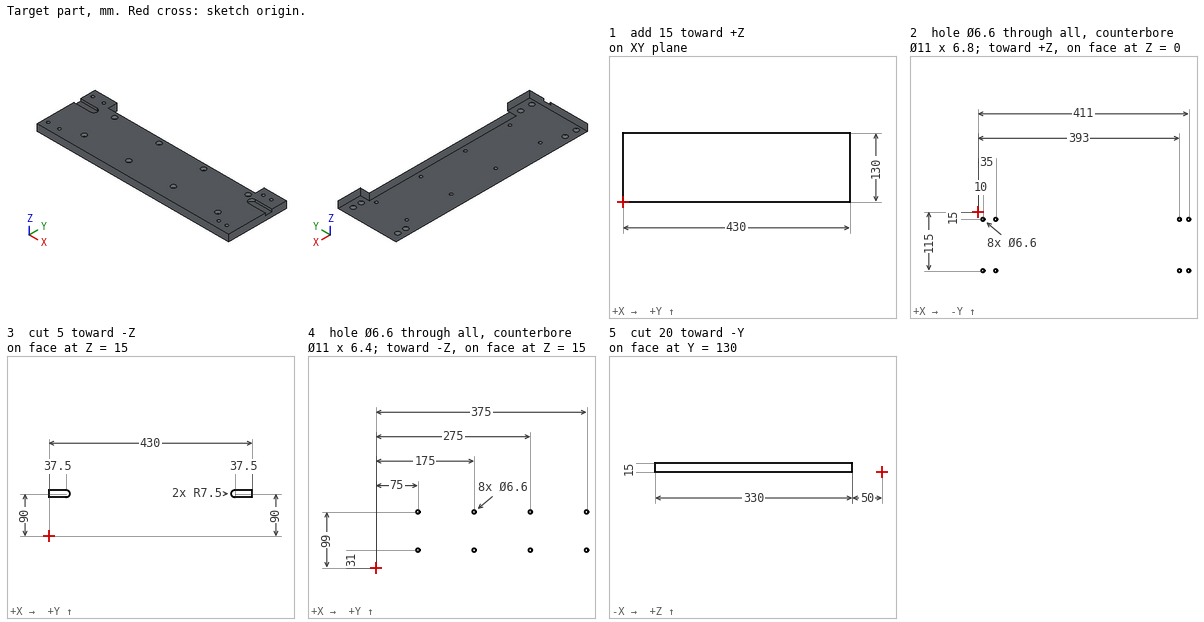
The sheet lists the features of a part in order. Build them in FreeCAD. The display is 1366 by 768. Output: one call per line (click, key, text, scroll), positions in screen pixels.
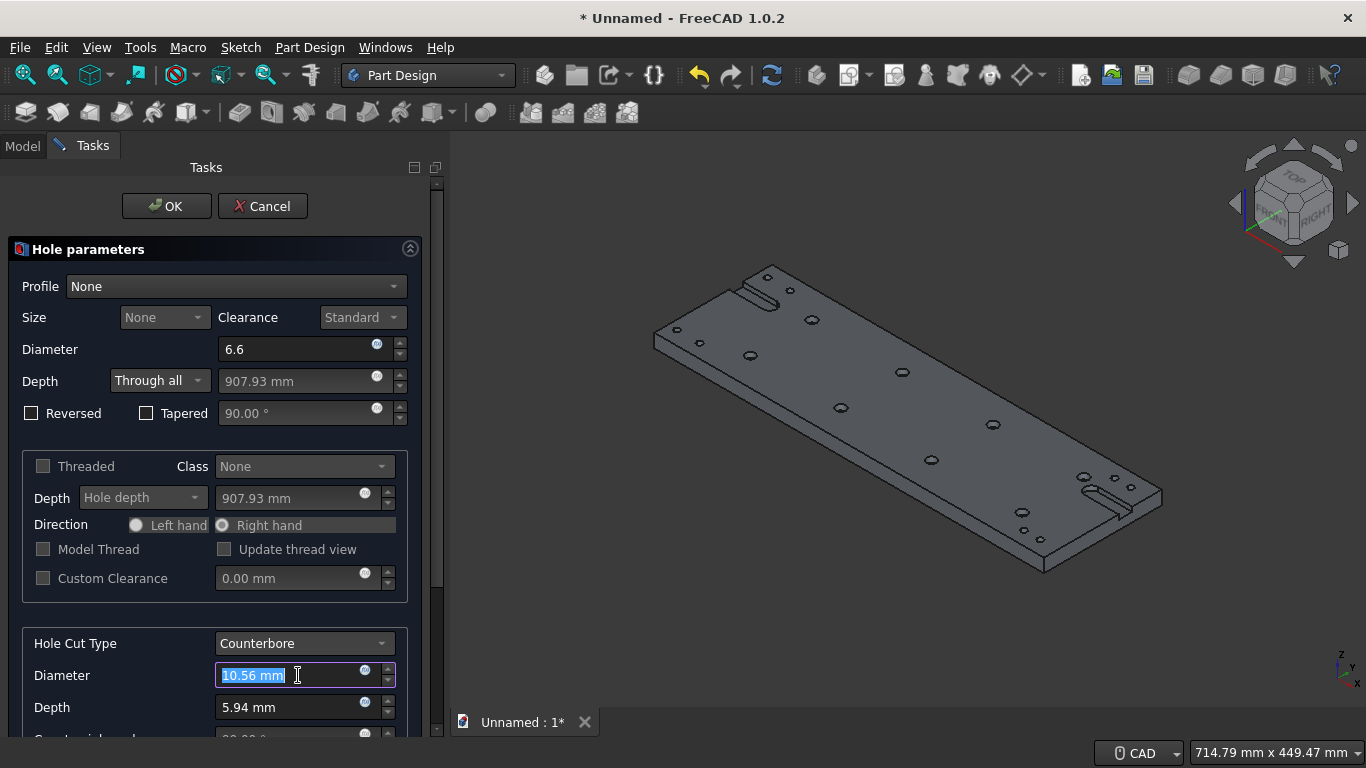
text(11)
key(Tab)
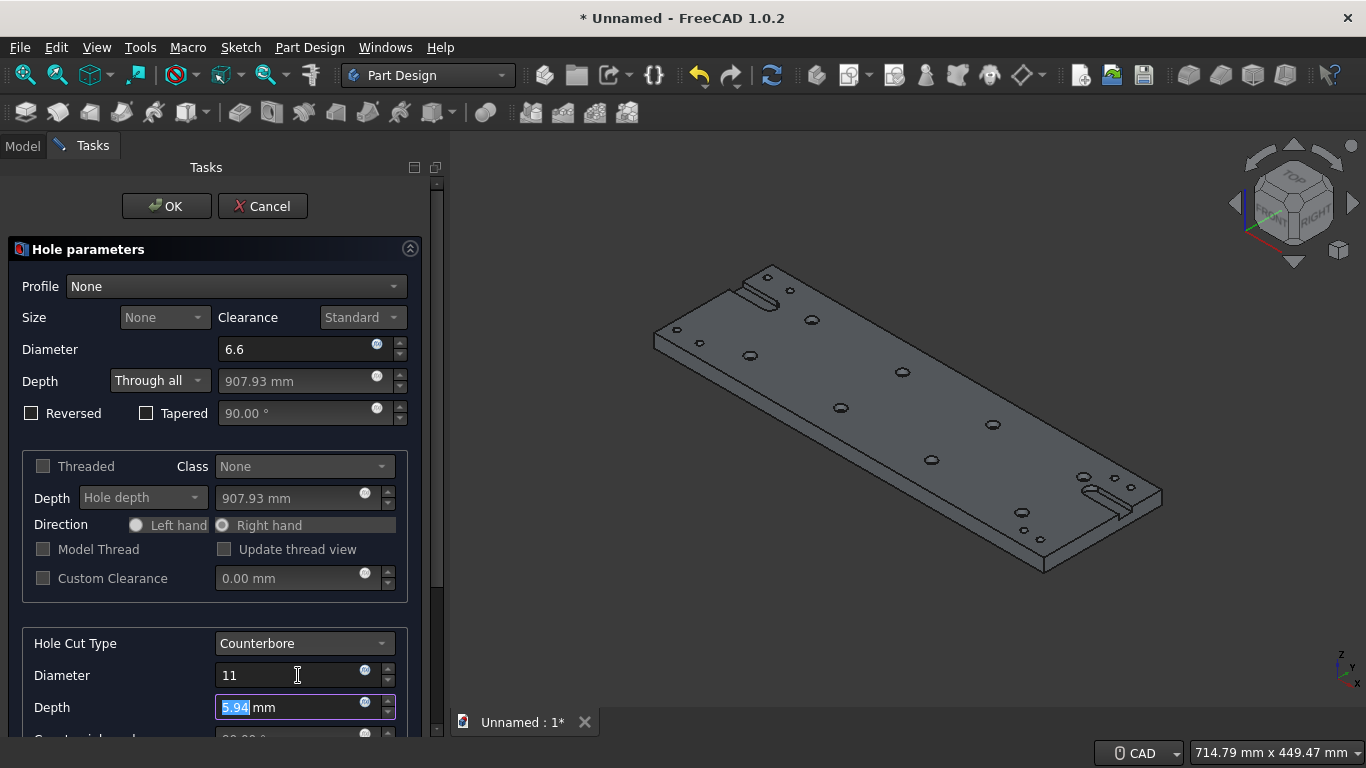
text(6.4)
key(Tab)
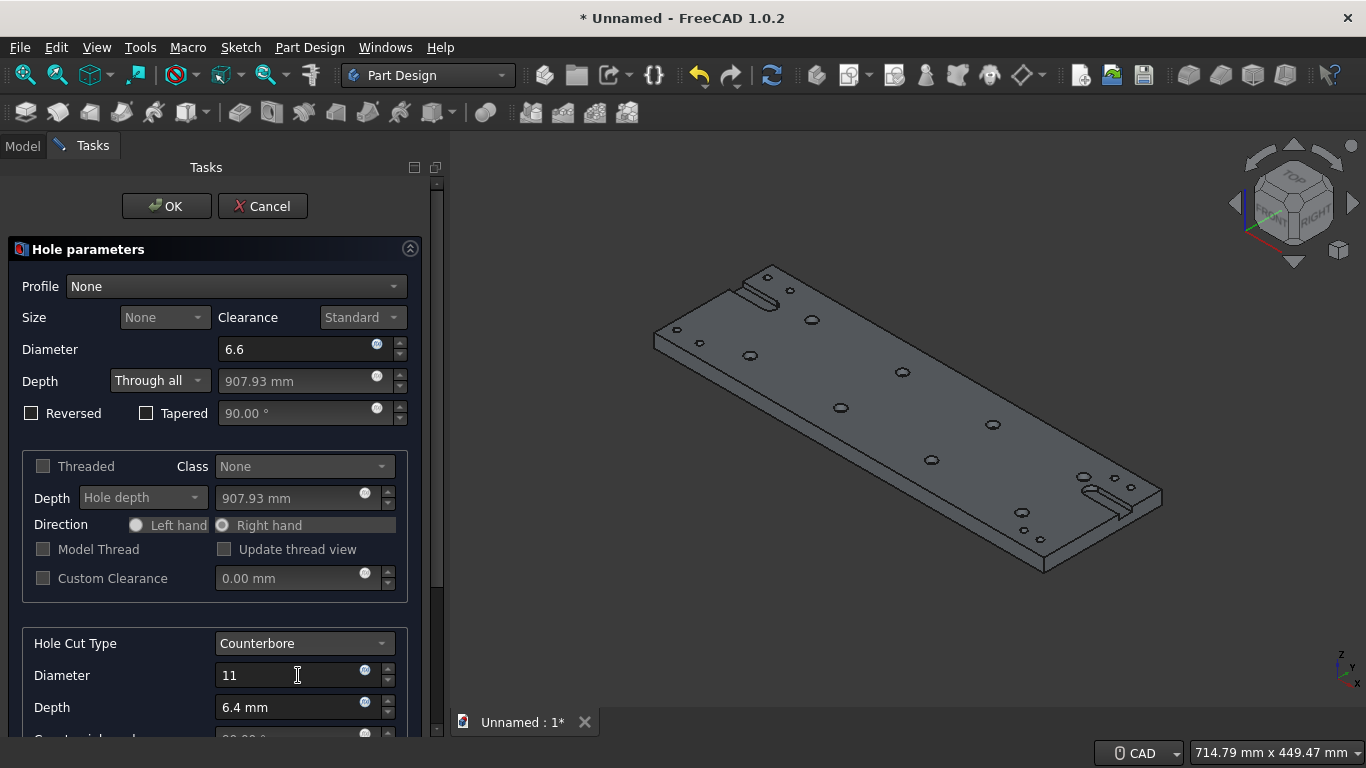
click(167, 206)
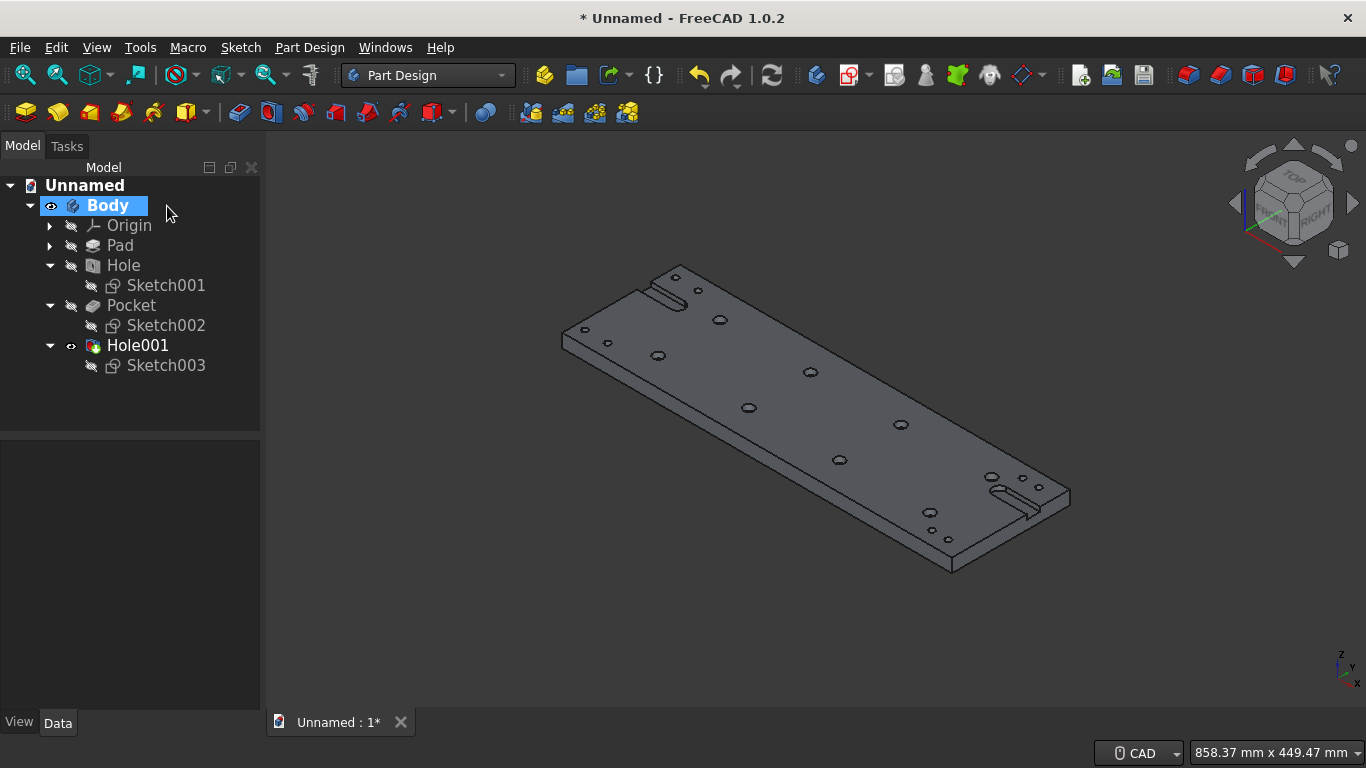
key(4)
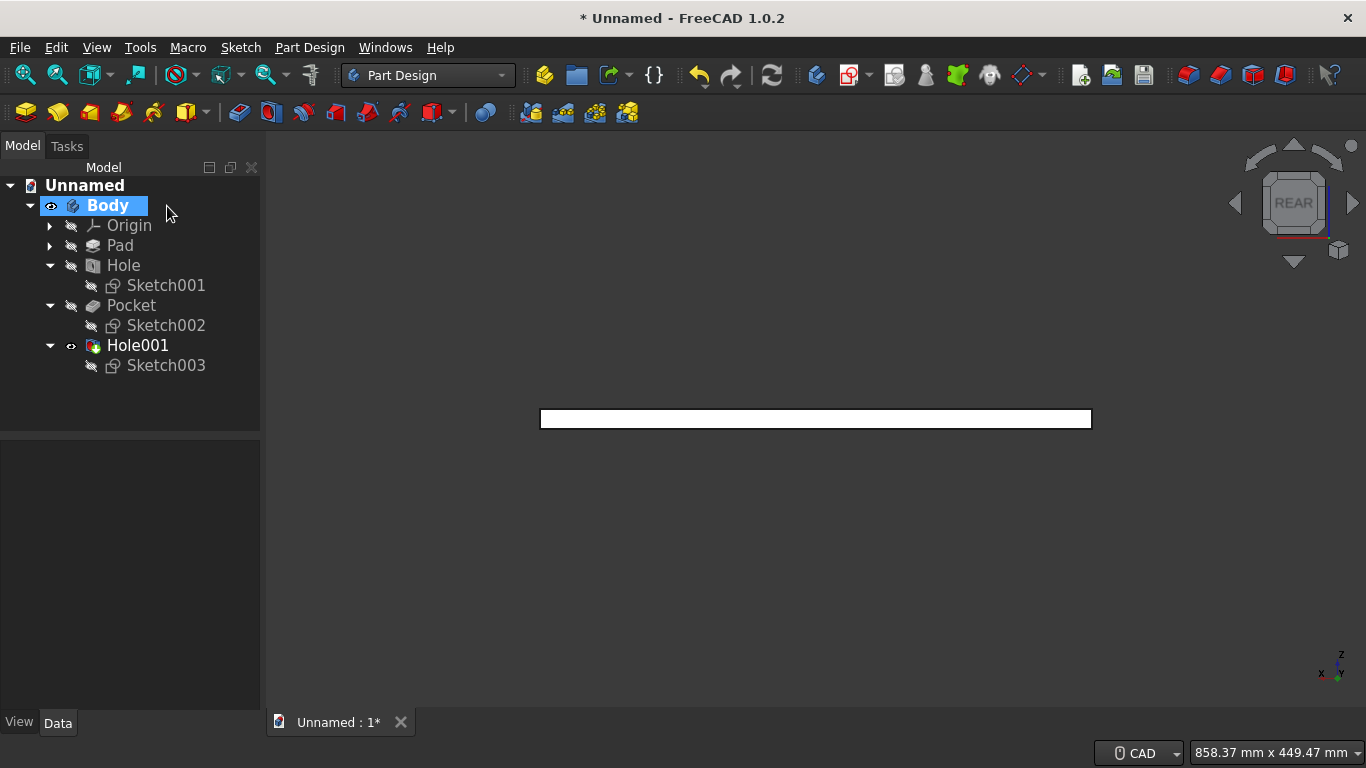
click(580, 418)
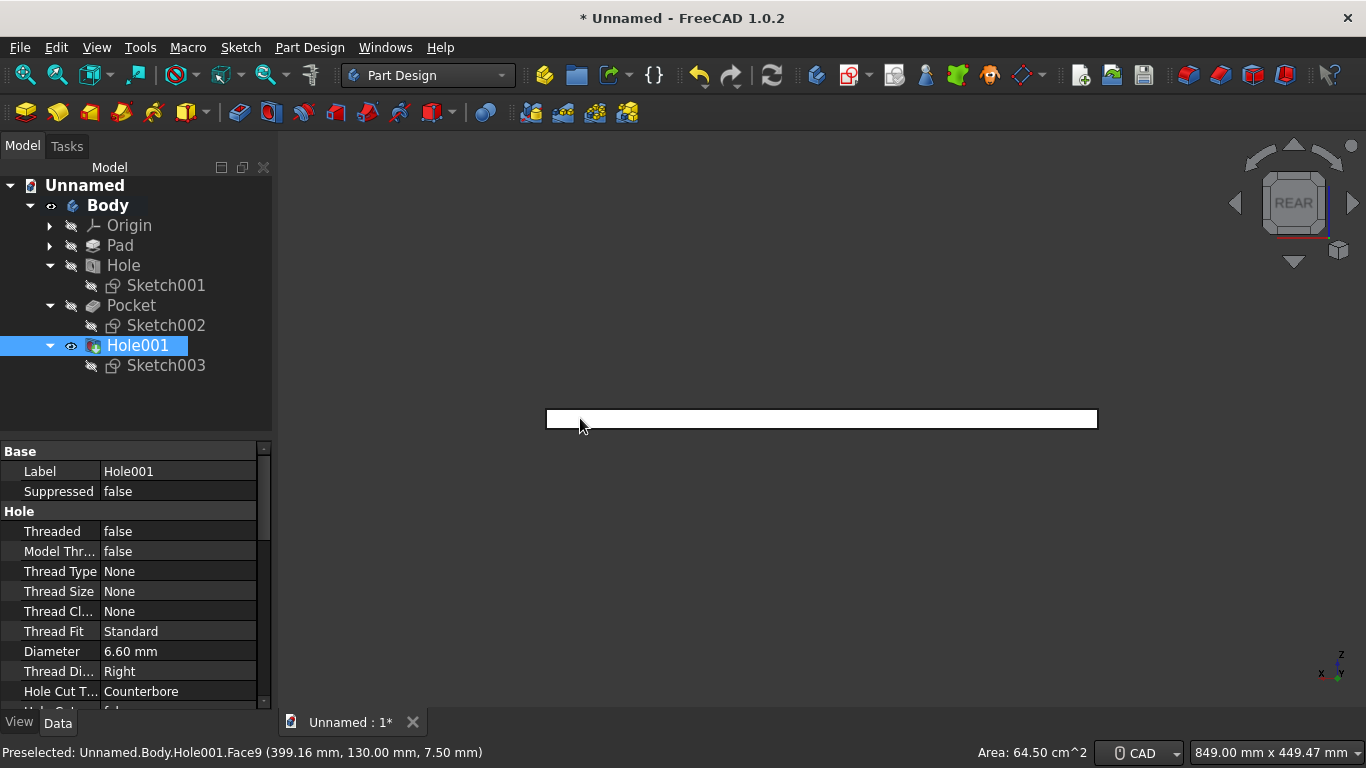
click(850, 76)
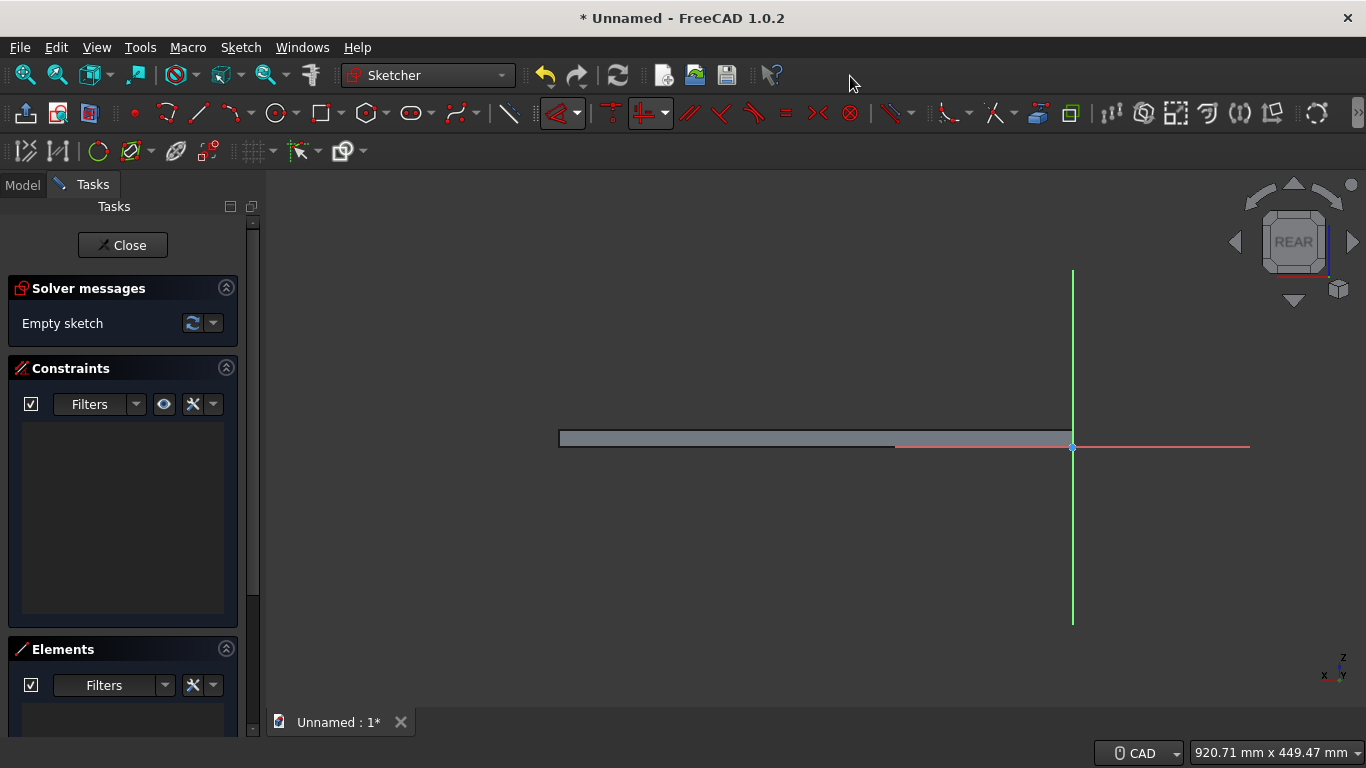
scroll(1046, 438, up, 2)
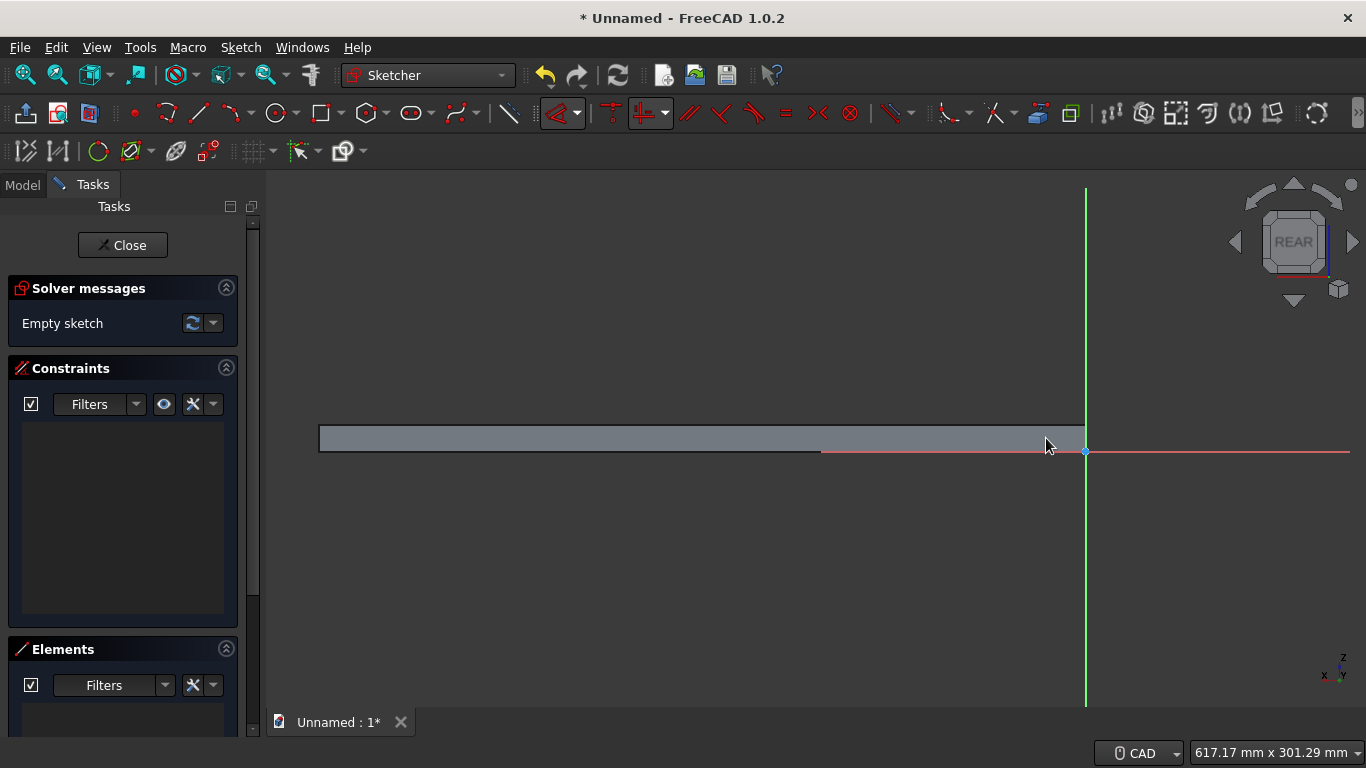
click(322, 114)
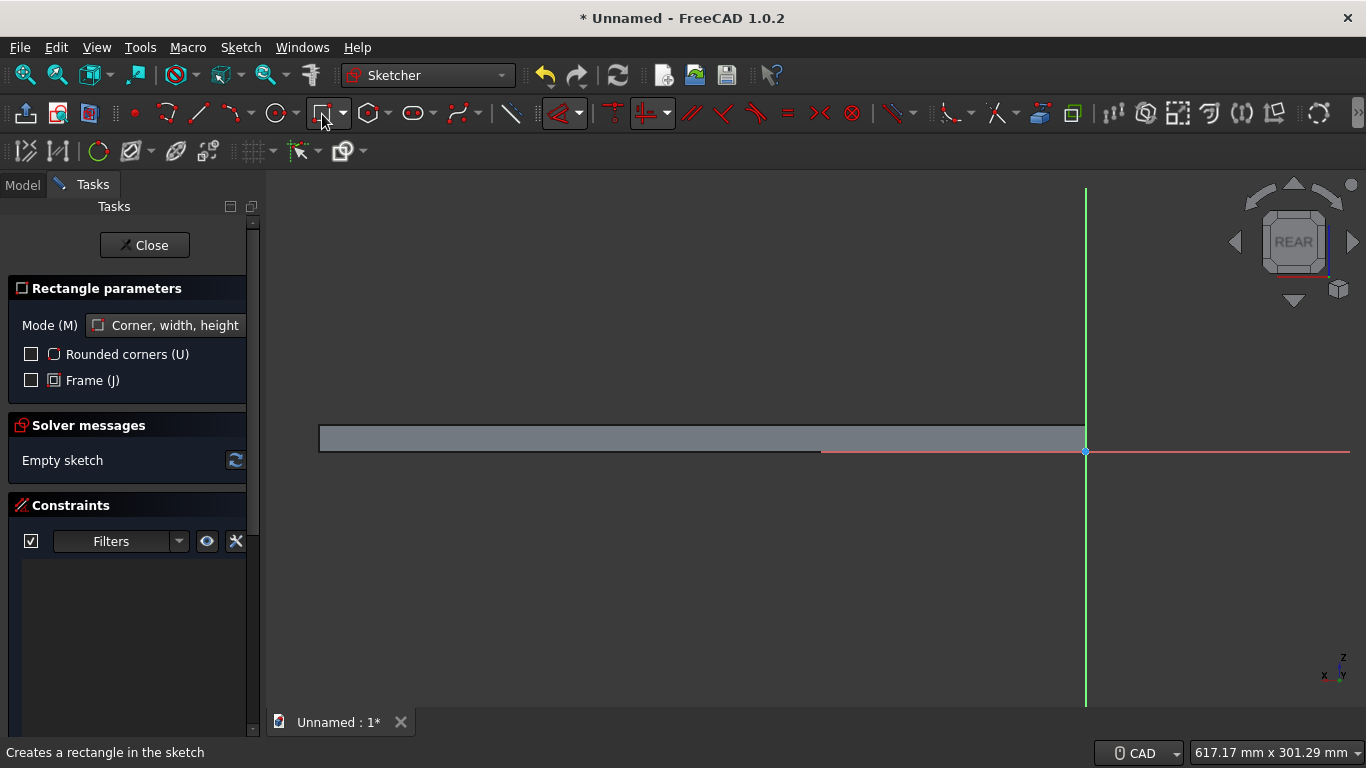
click(408, 425)
click(997, 452)
key(Escape)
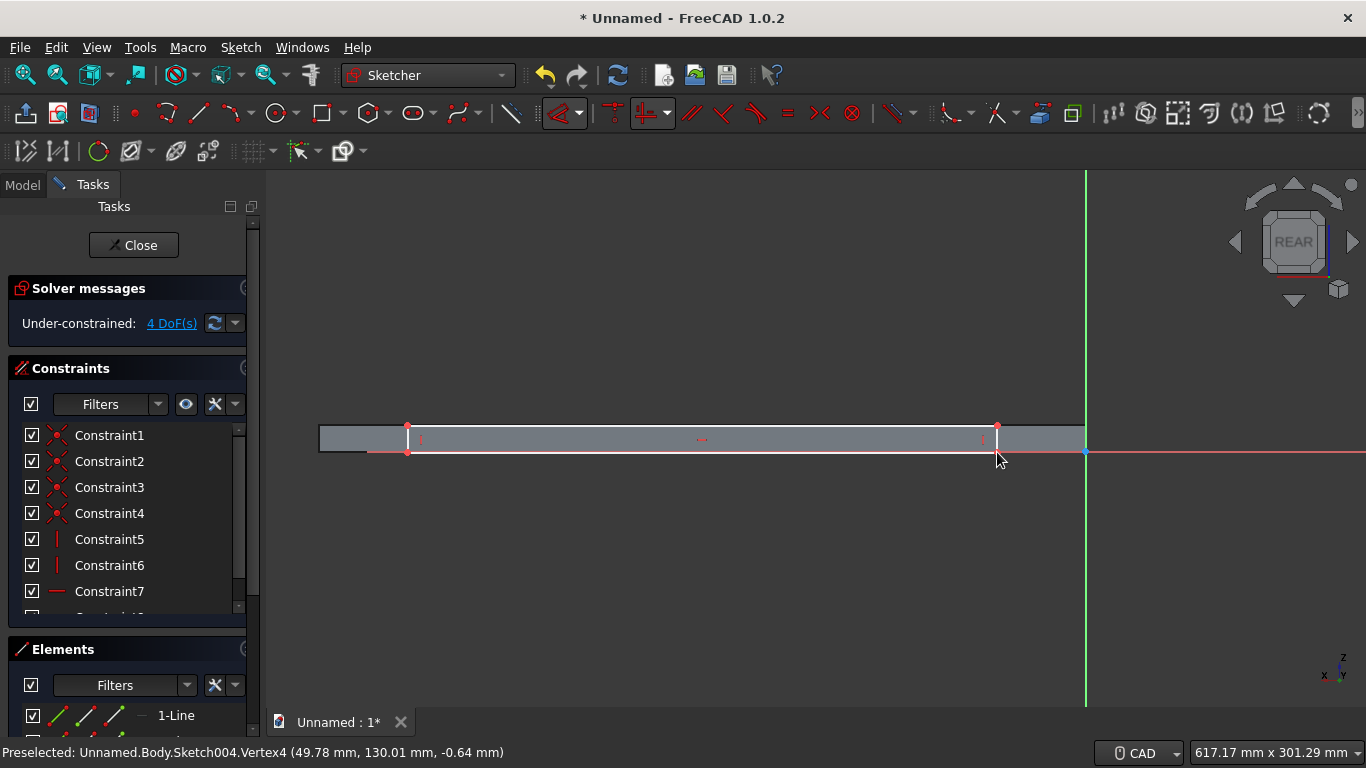
click(408, 453)